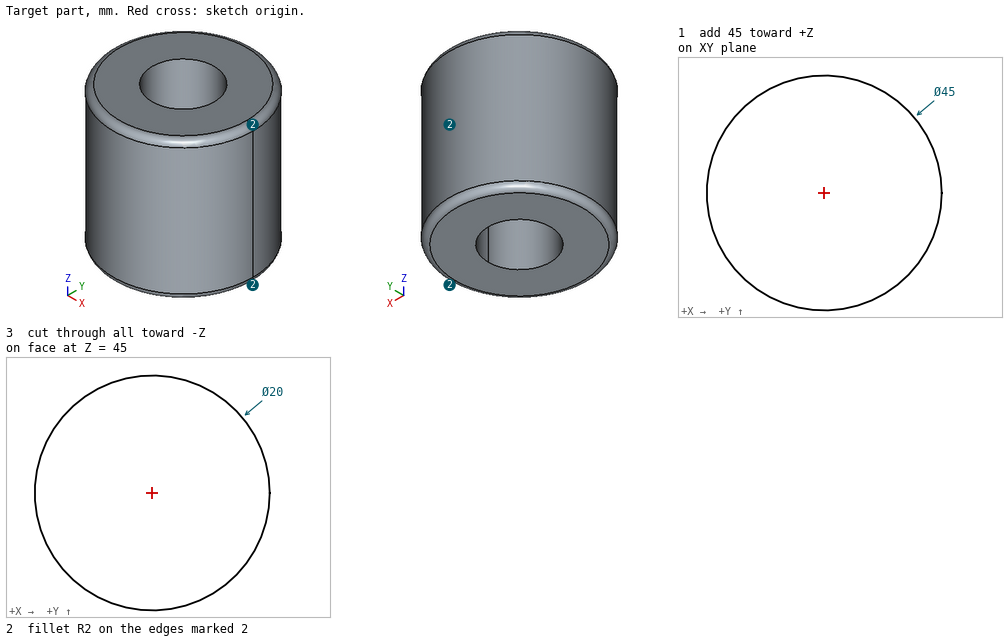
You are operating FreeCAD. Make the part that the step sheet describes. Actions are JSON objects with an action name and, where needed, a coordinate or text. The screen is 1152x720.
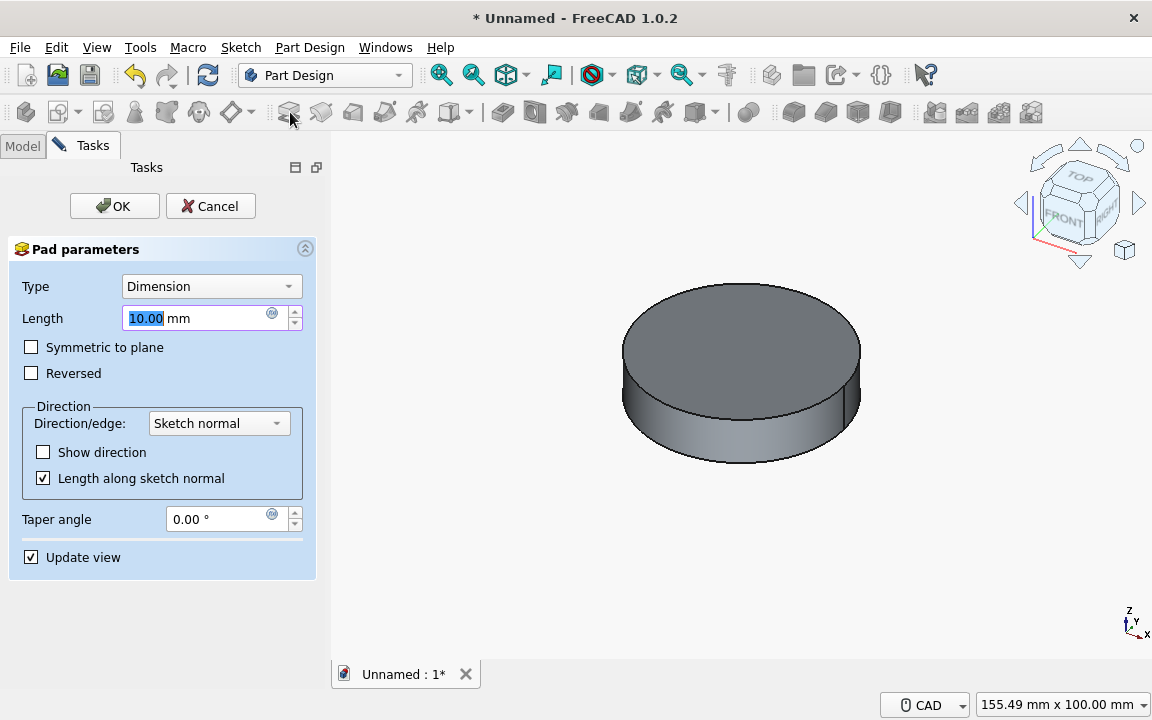
{"action": "type", "text": "45"}
{"action": "key", "text": "Tab"}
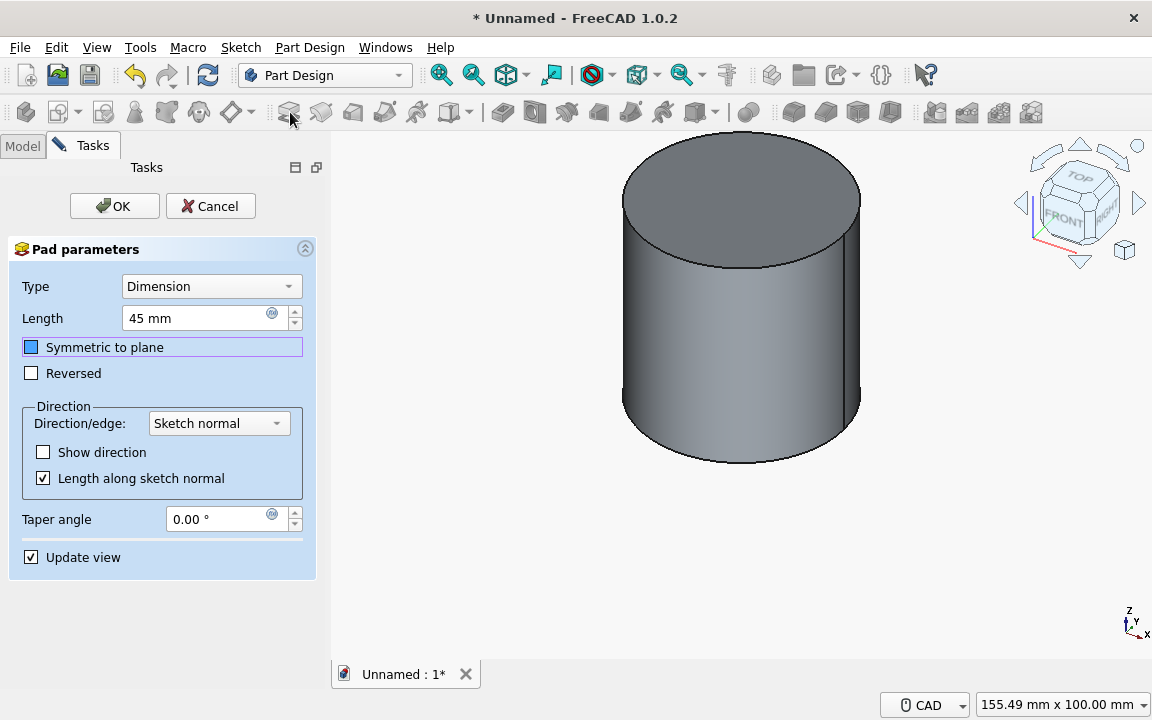
{"action": "left_click", "coordinate": [115, 206]}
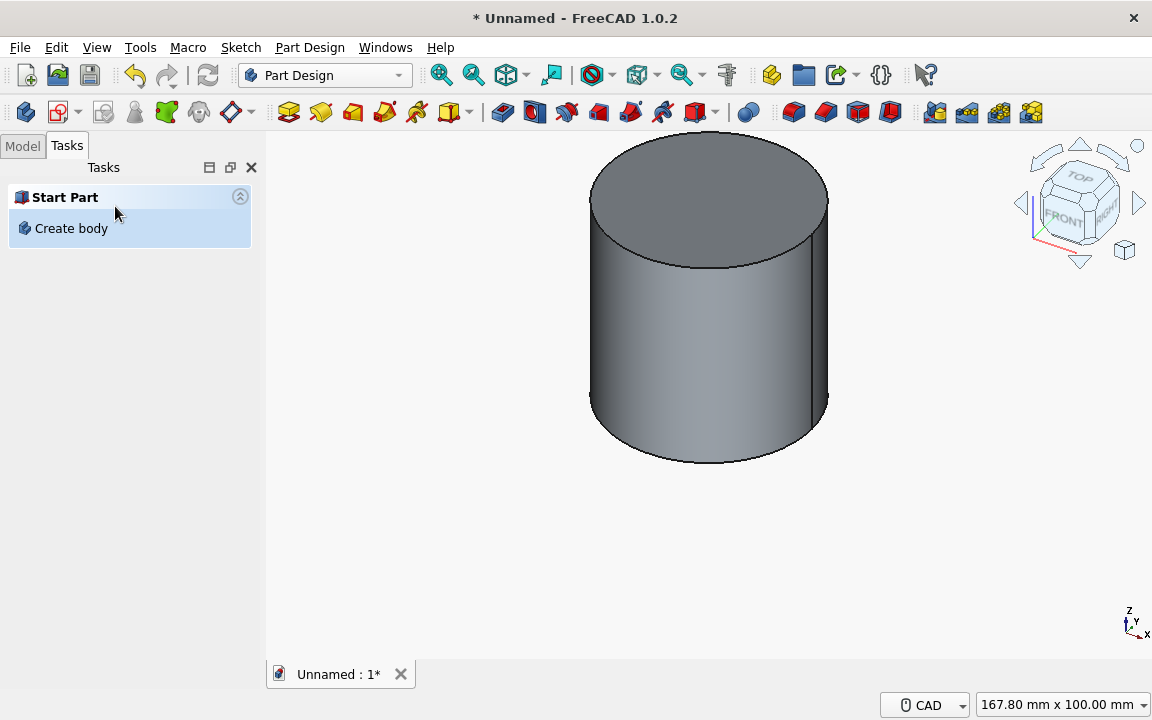
{"action": "left_click", "coordinate": [442, 76]}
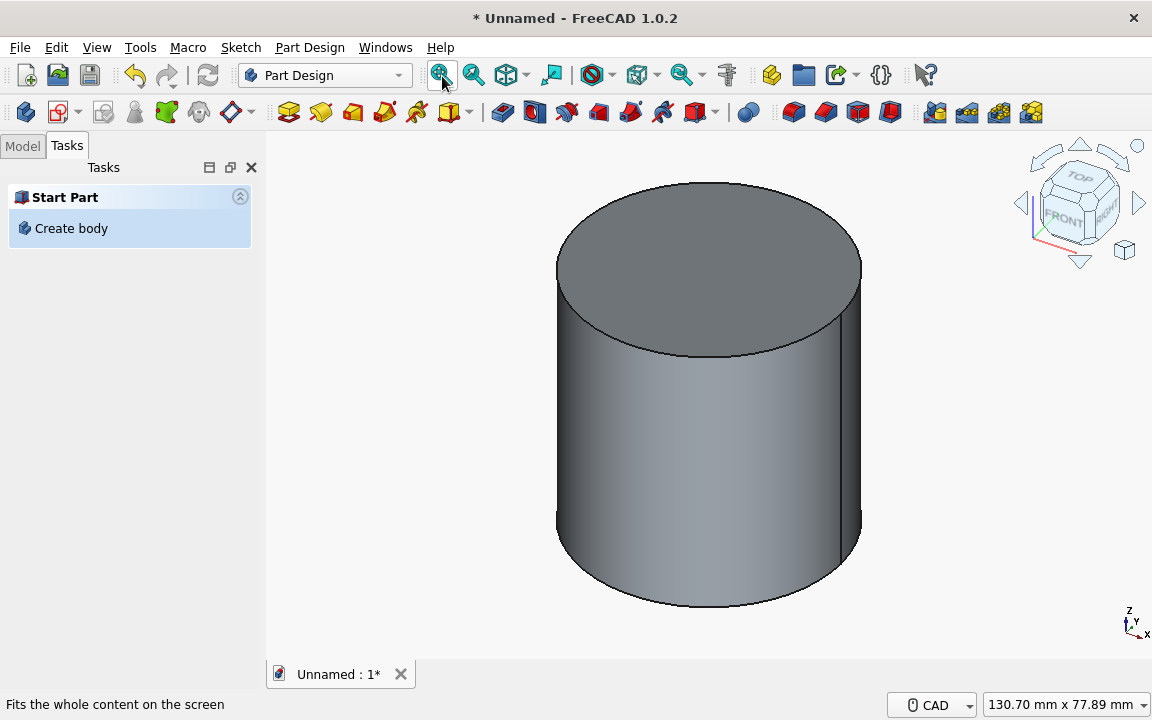
{"action": "left_click", "coordinate": [557, 278]}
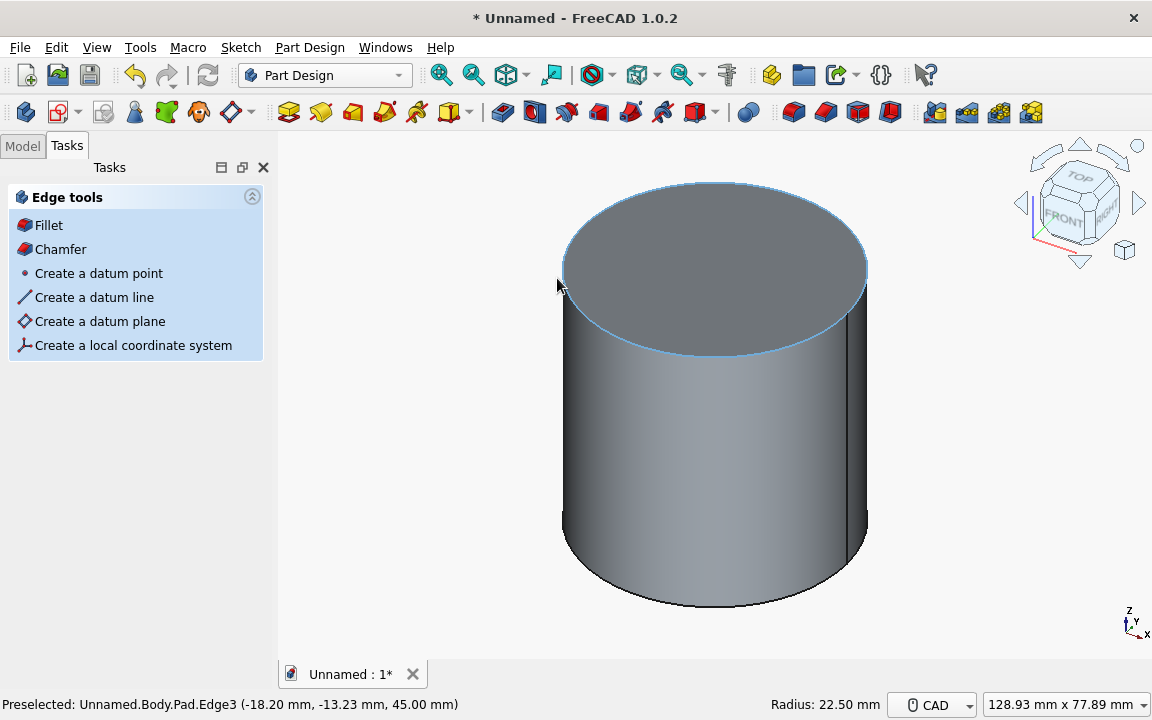
{"action": "key", "text": "0"}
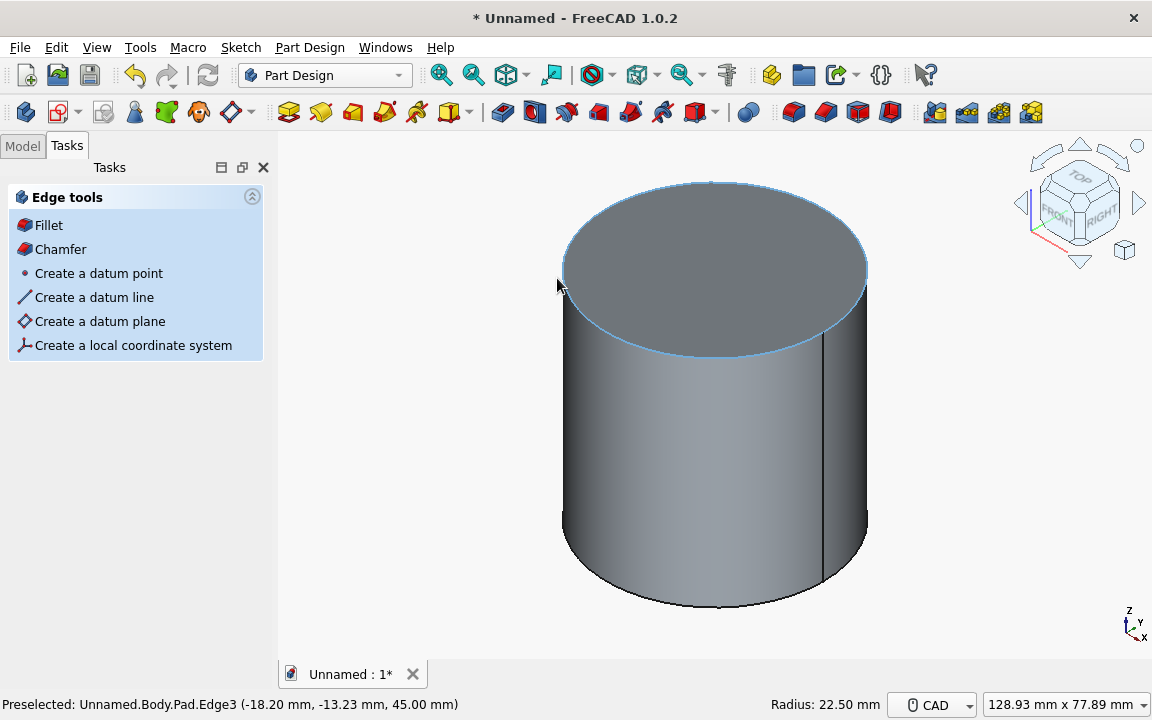
{"action": "key", "text": "2"}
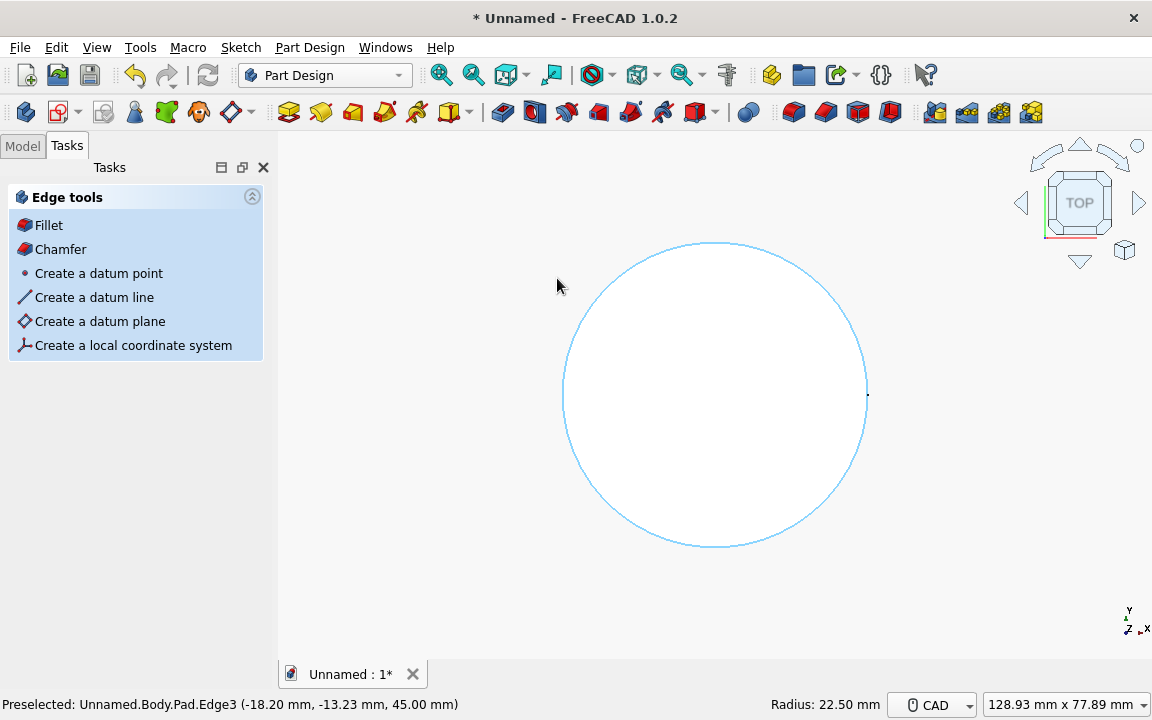
{"action": "key", "text": "1"}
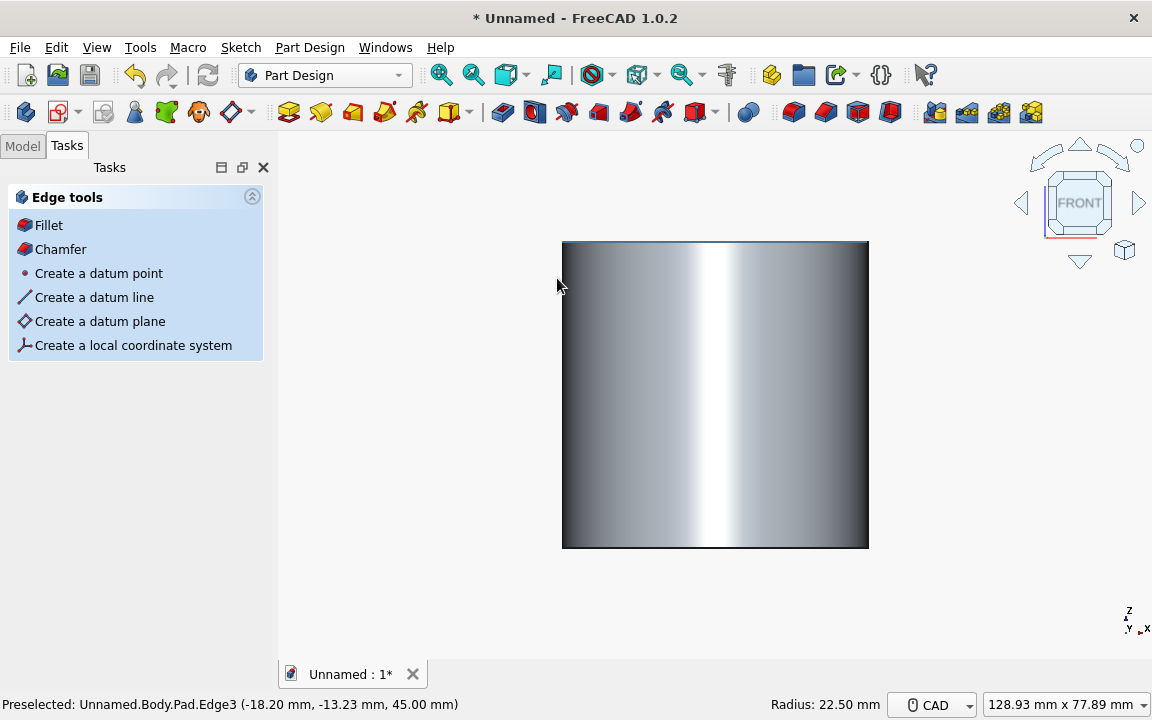
{"action": "left_click", "coordinate": [592, 547], "text": "ctrl"}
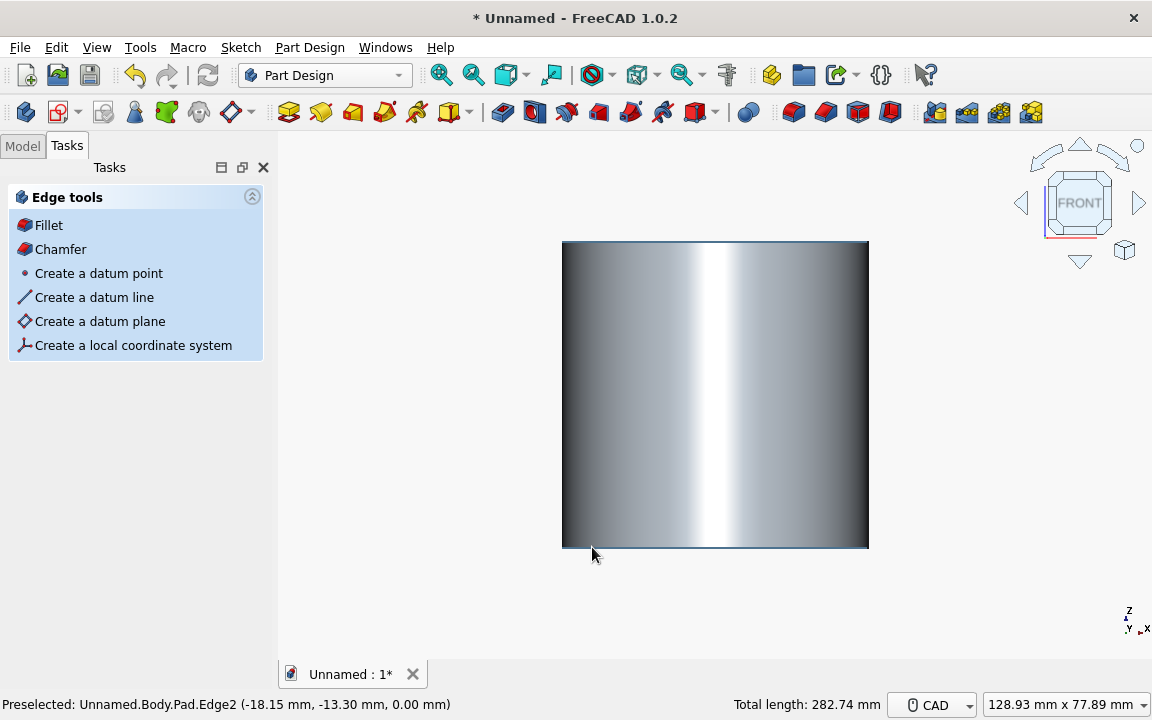
{"action": "left_click", "coordinate": [794, 112]}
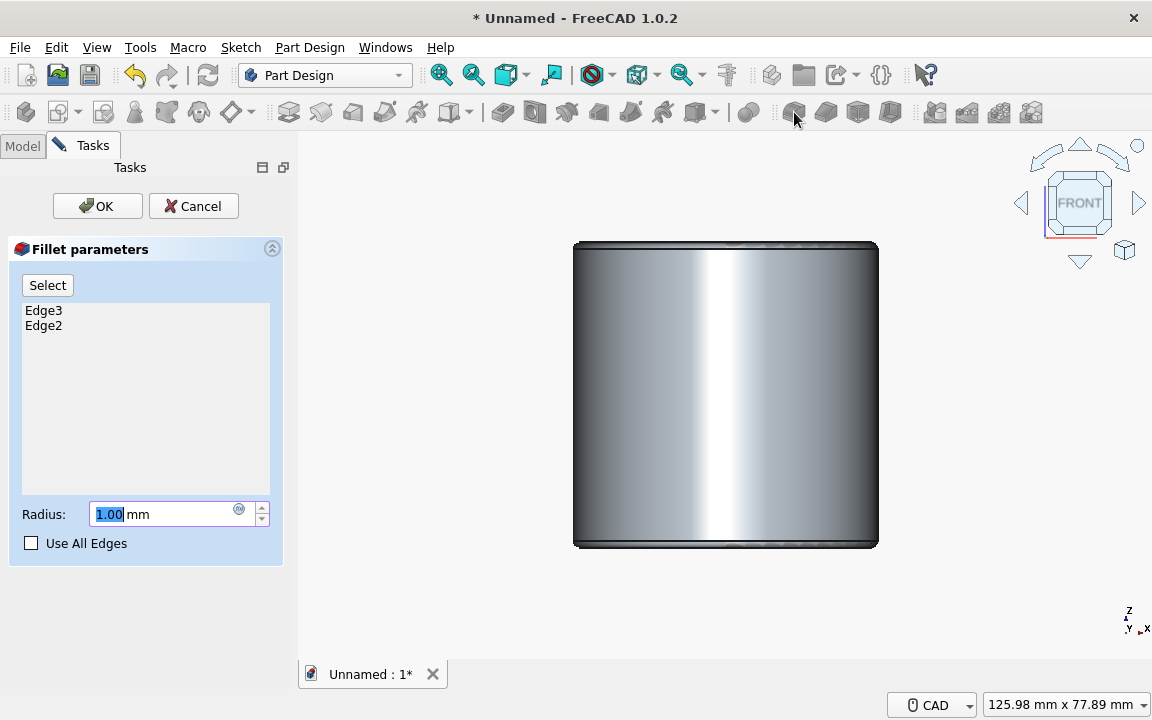
{"action": "type", "text": "2"}
{"action": "key", "text": "Tab"}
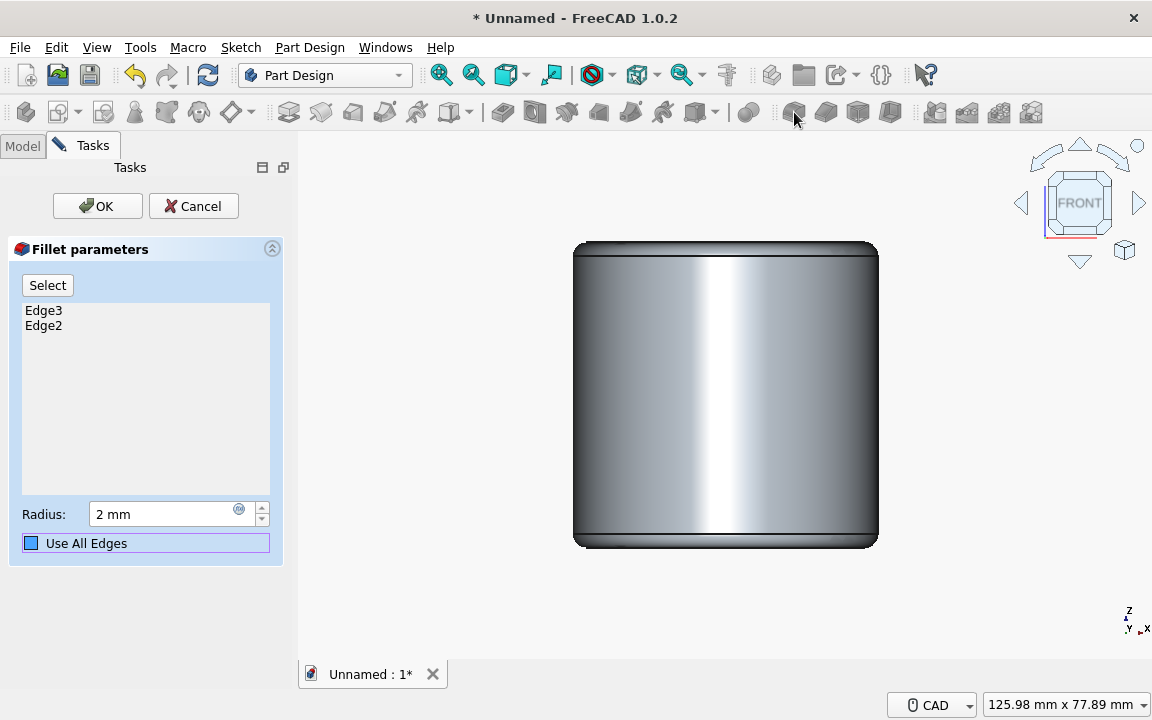
{"action": "left_click", "coordinate": [98, 206]}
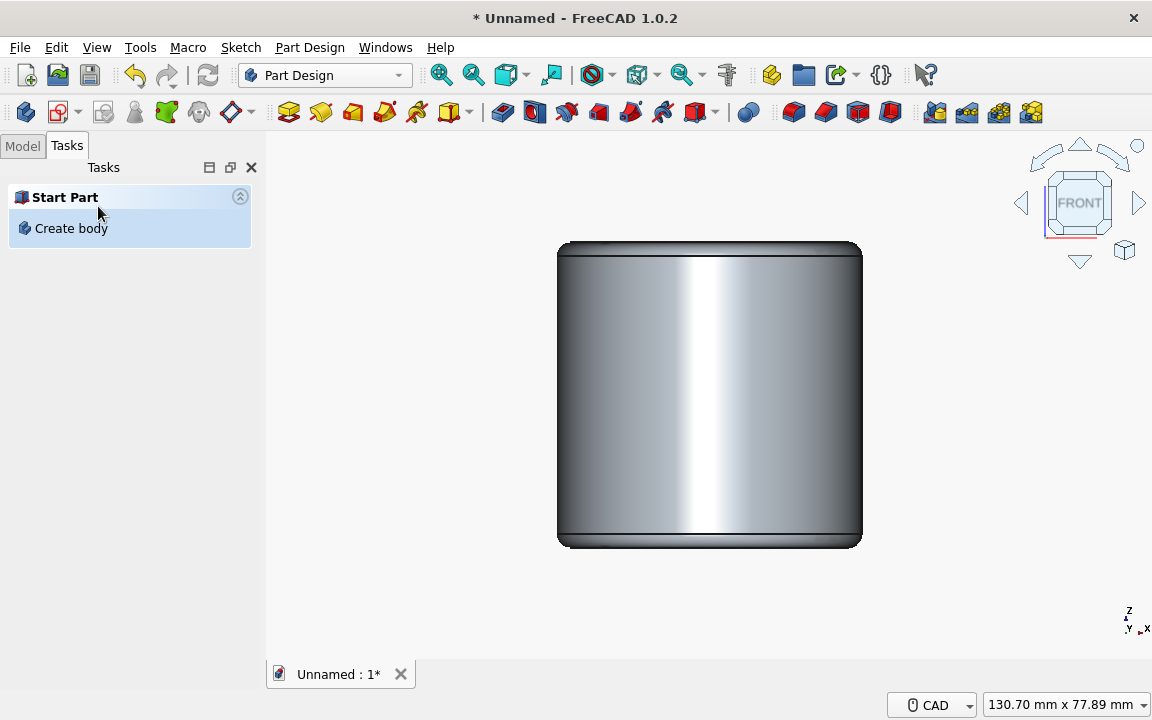
{"action": "key", "text": "0"}